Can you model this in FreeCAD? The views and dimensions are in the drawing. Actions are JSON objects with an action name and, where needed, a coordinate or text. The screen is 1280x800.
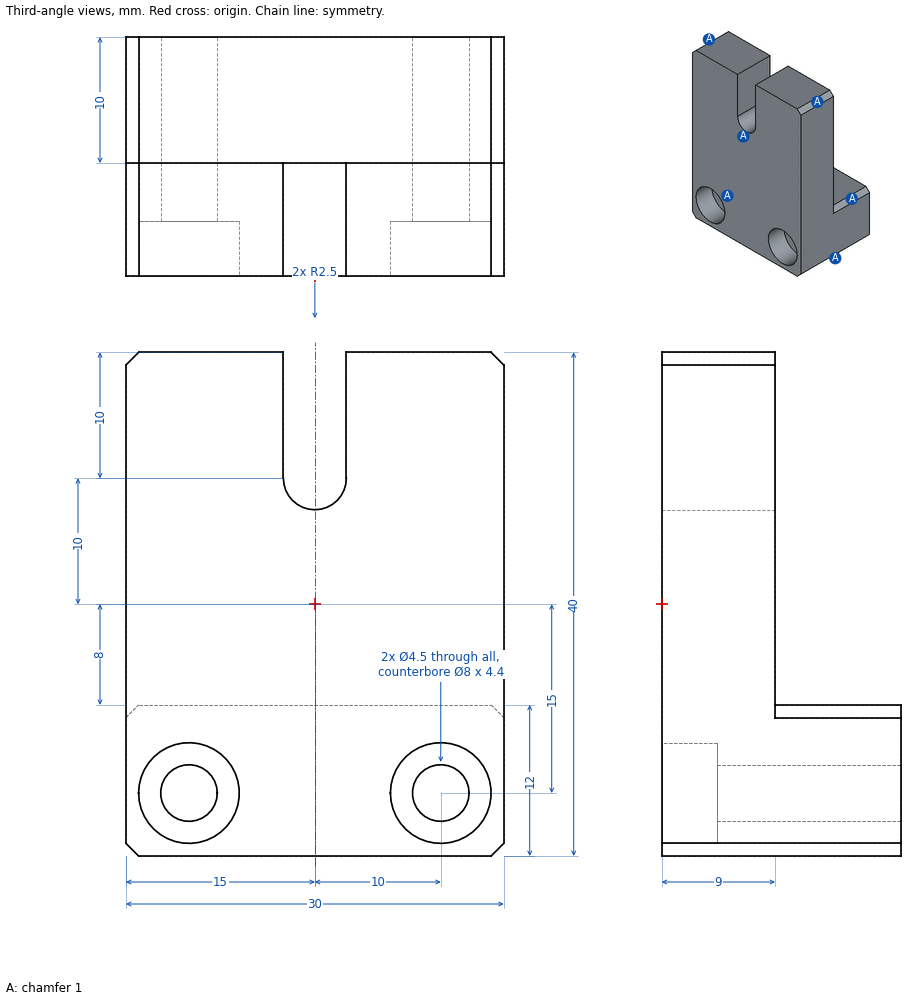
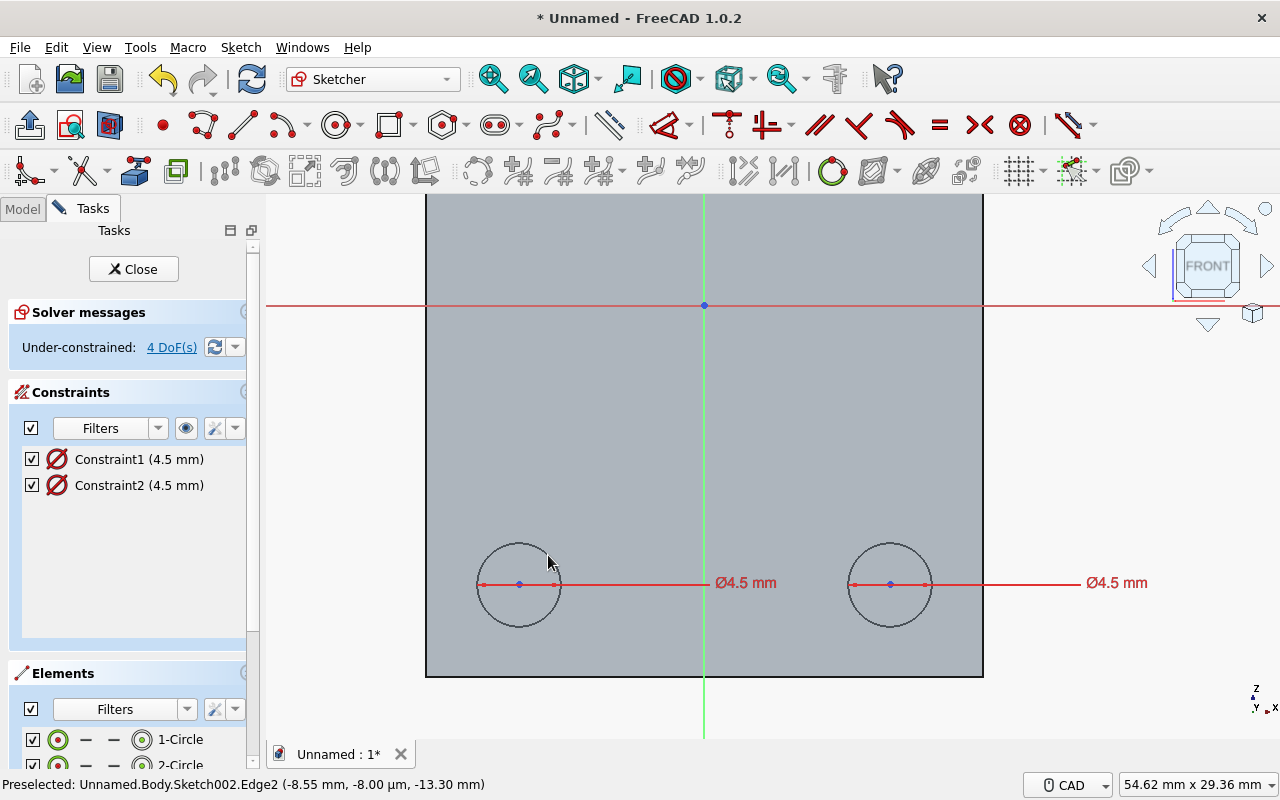
{"action": "left_click", "coordinate": [890, 585]}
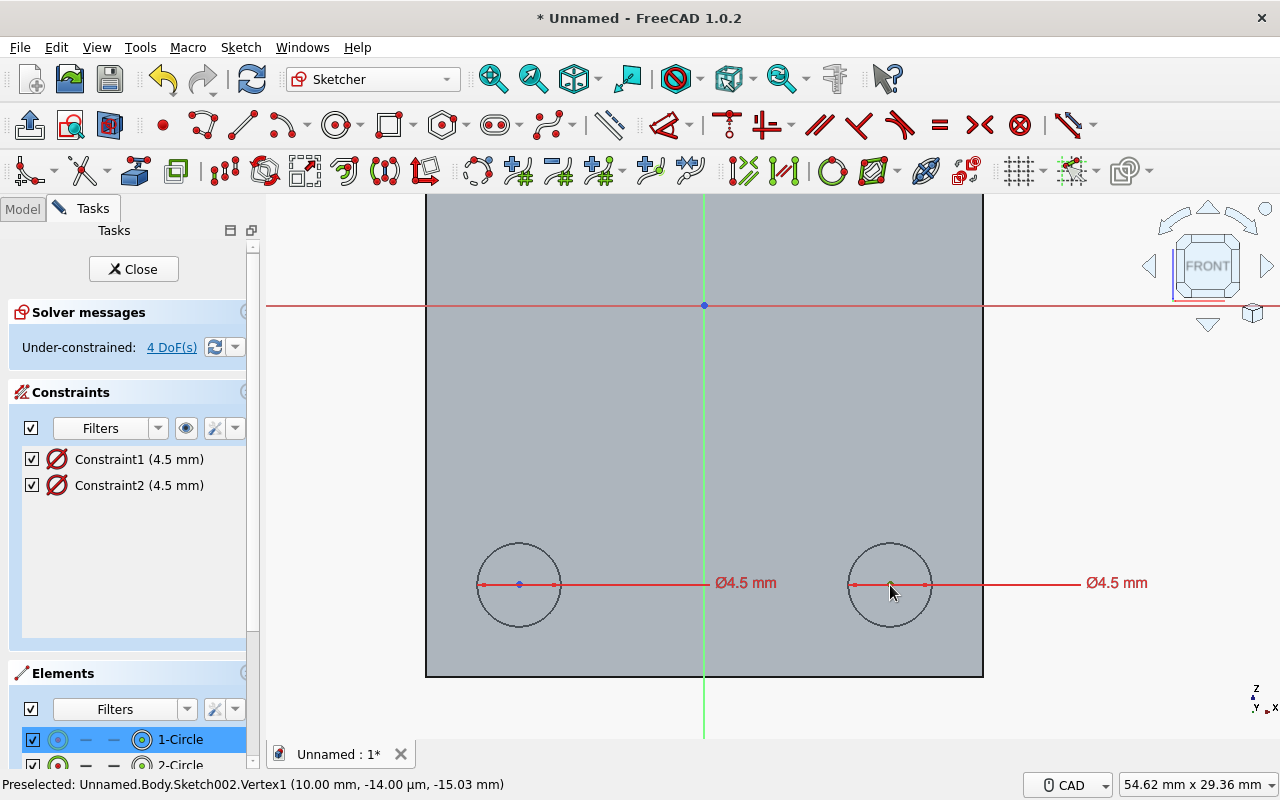
{"action": "left_click", "coordinate": [519, 585]}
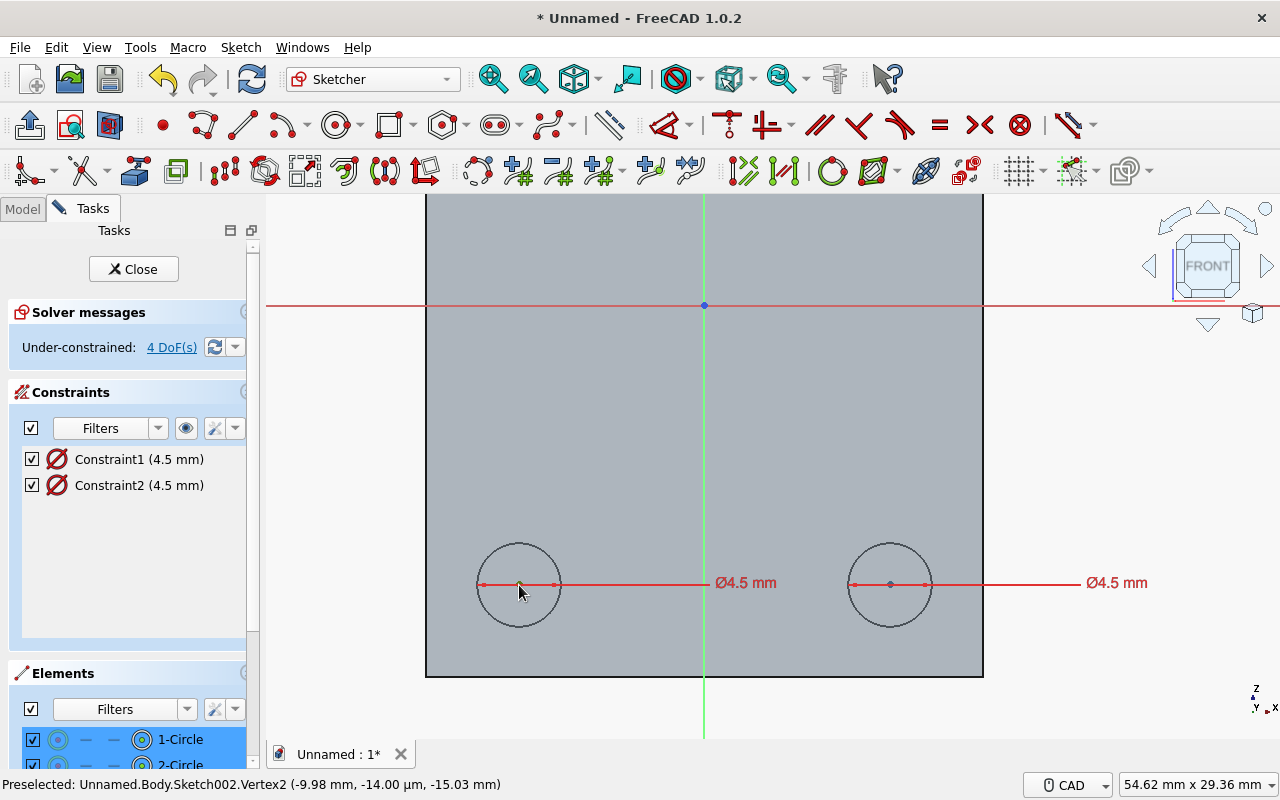
{"action": "left_click", "coordinate": [704, 676]}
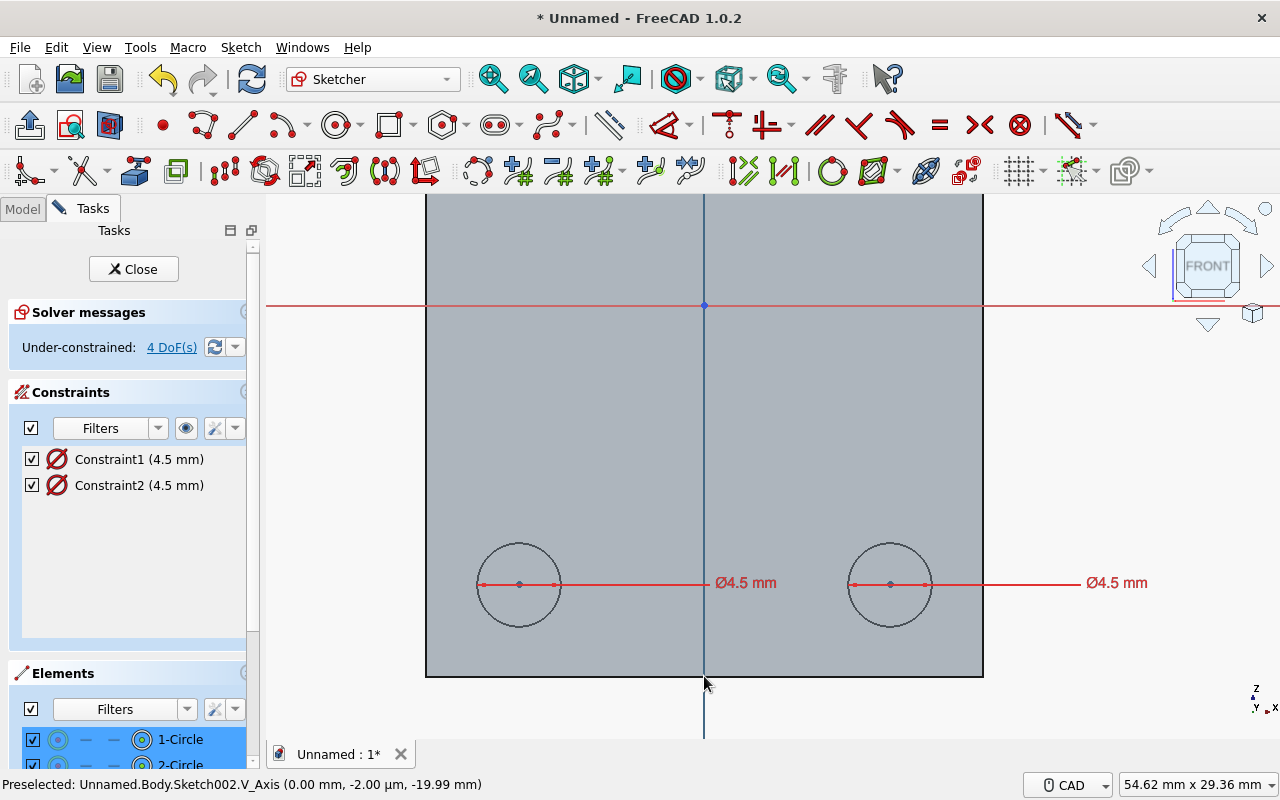
{"action": "left_click", "coordinate": [980, 126]}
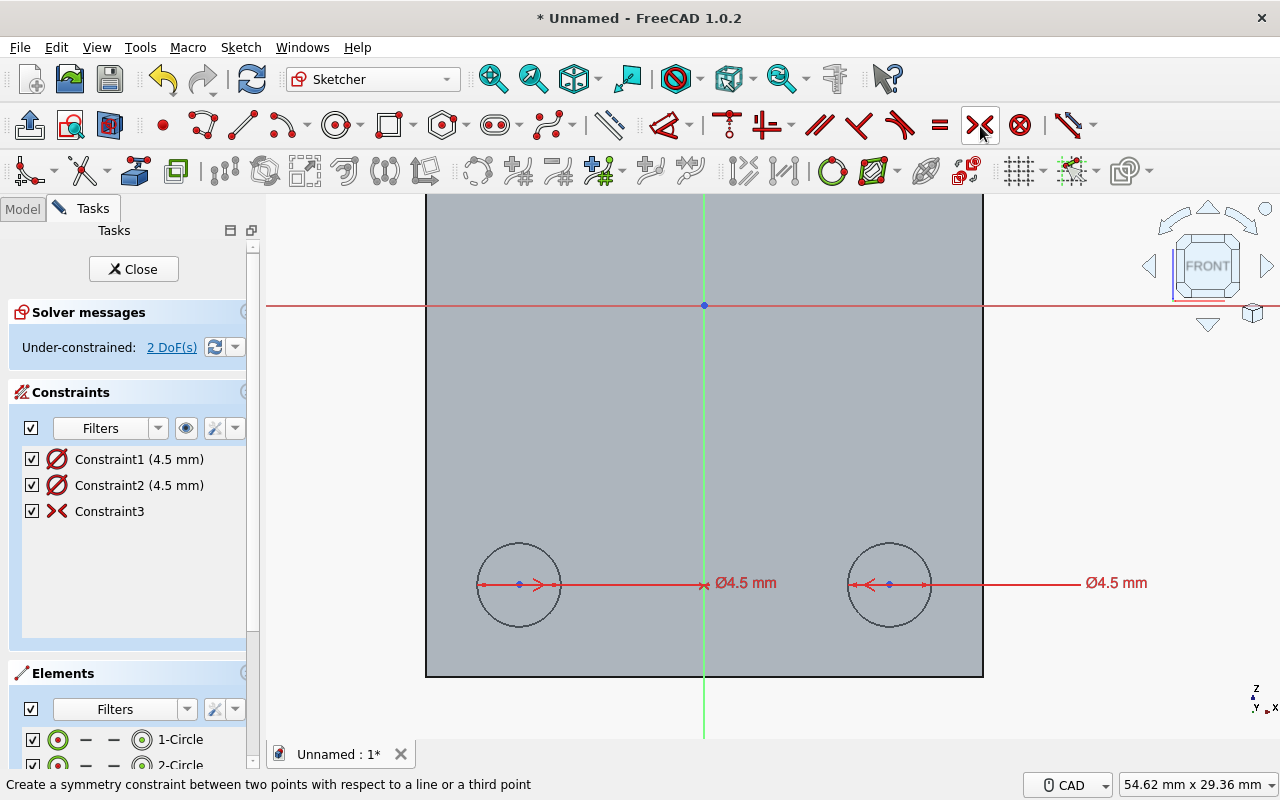
{"action": "left_click", "coordinate": [664, 126]}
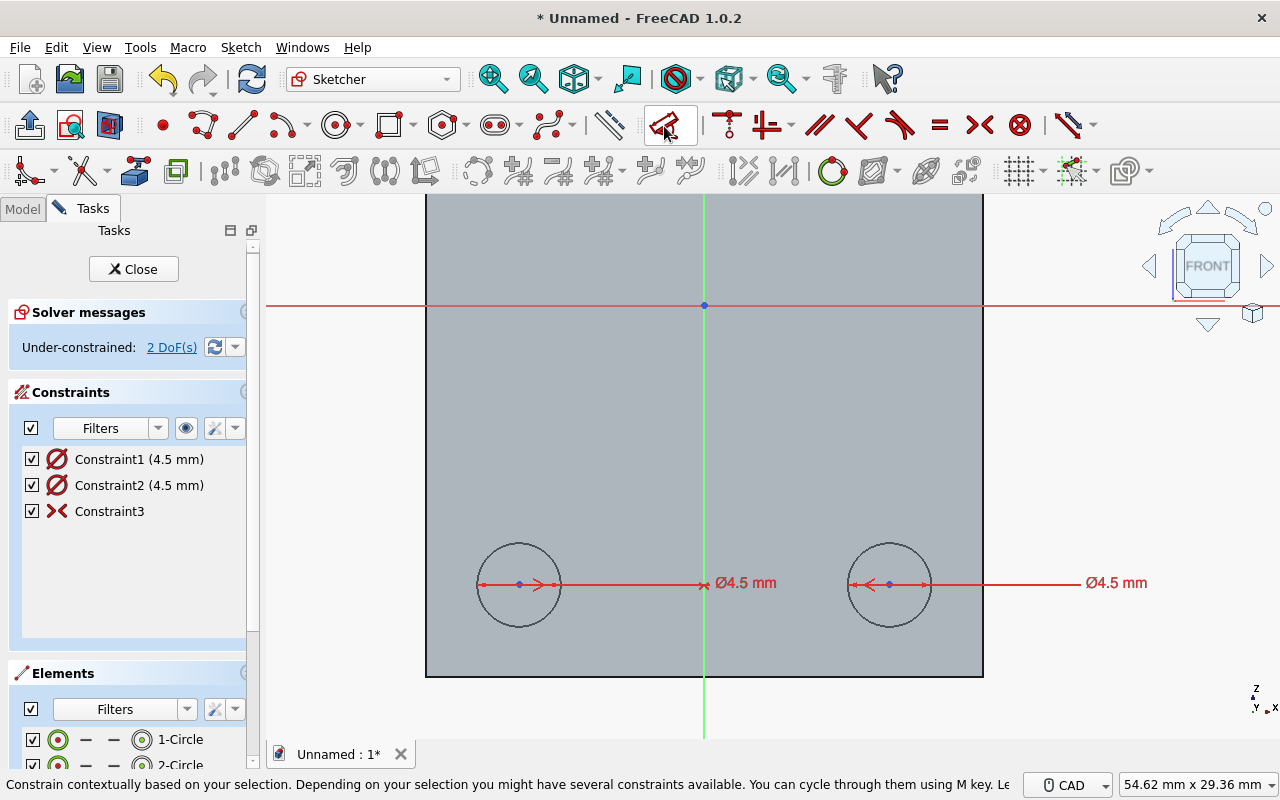
{"action": "left_click", "coordinate": [890, 585]}
{"action": "left_click", "coordinate": [797, 272]}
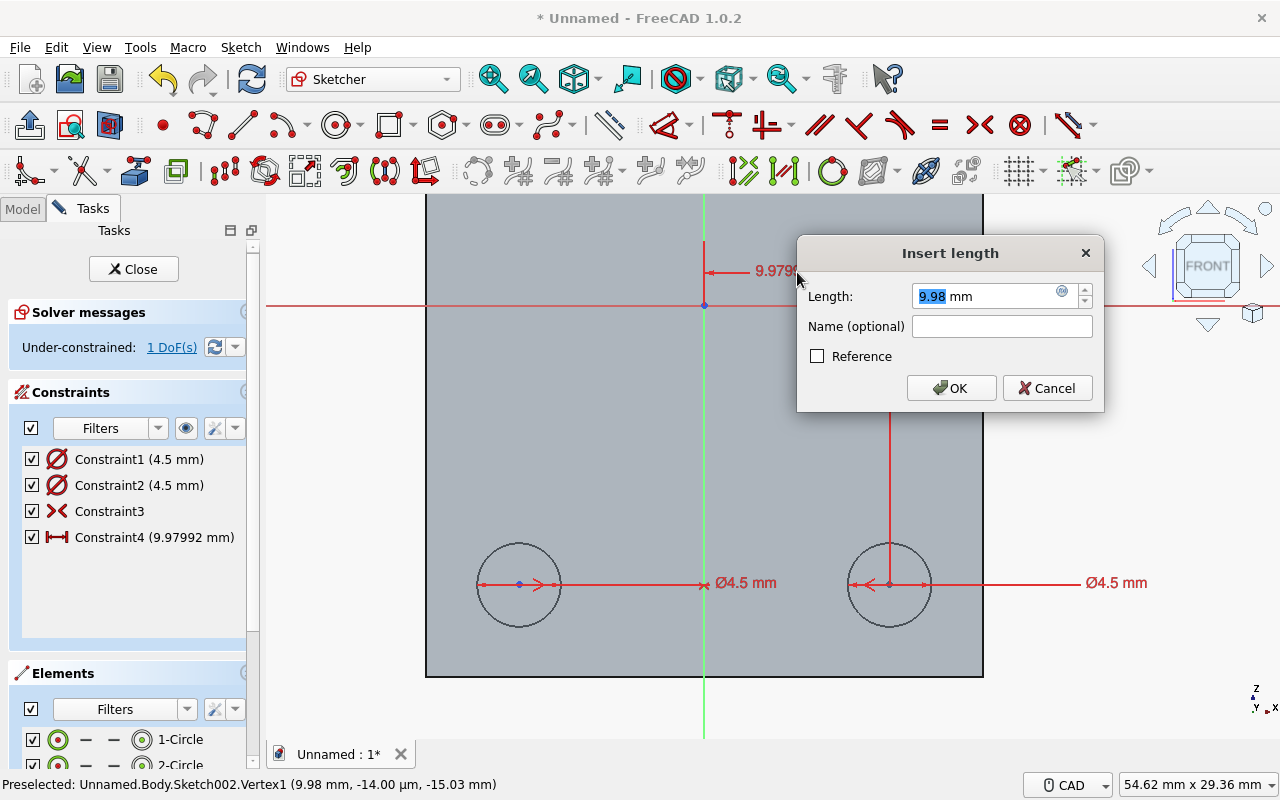
{"action": "type", "text": "10"}
{"action": "key", "text": "Return"}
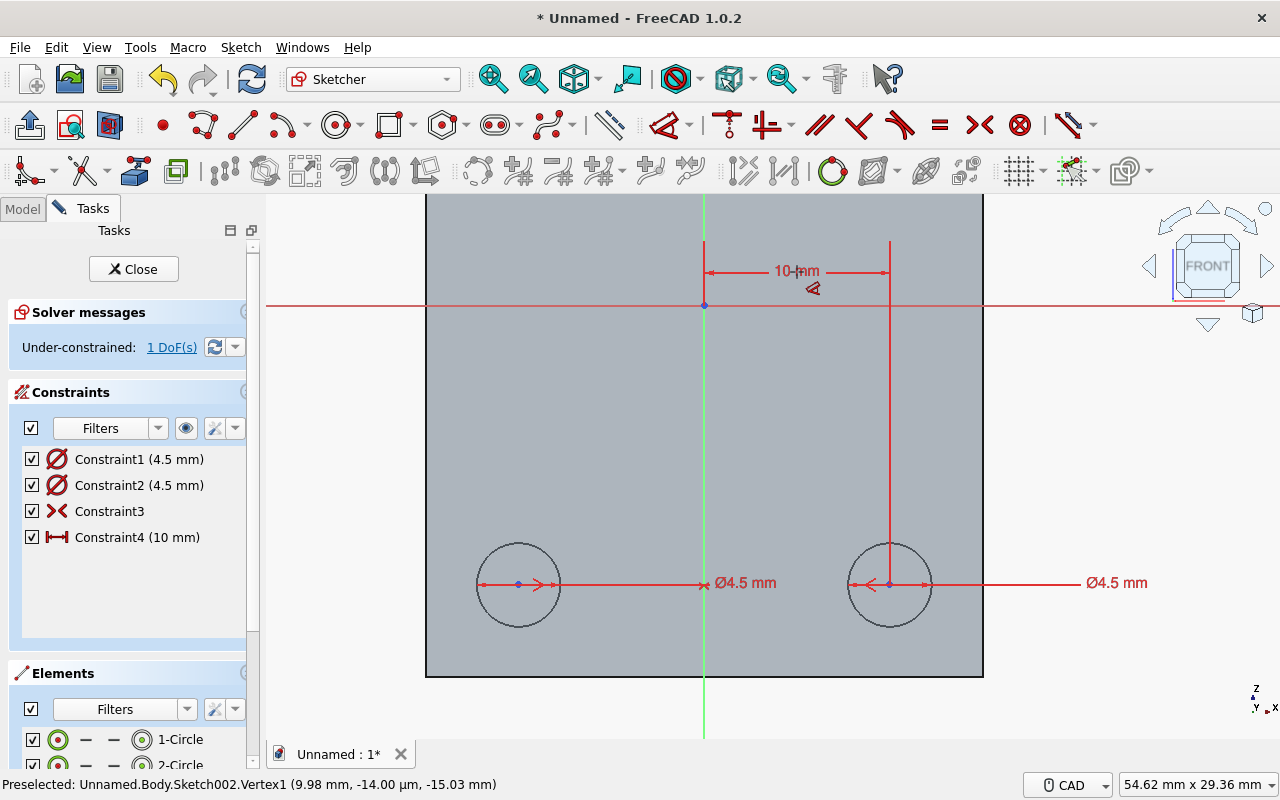
{"action": "left_click", "coordinate": [890, 585]}
{"action": "left_click", "coordinate": [924, 445]}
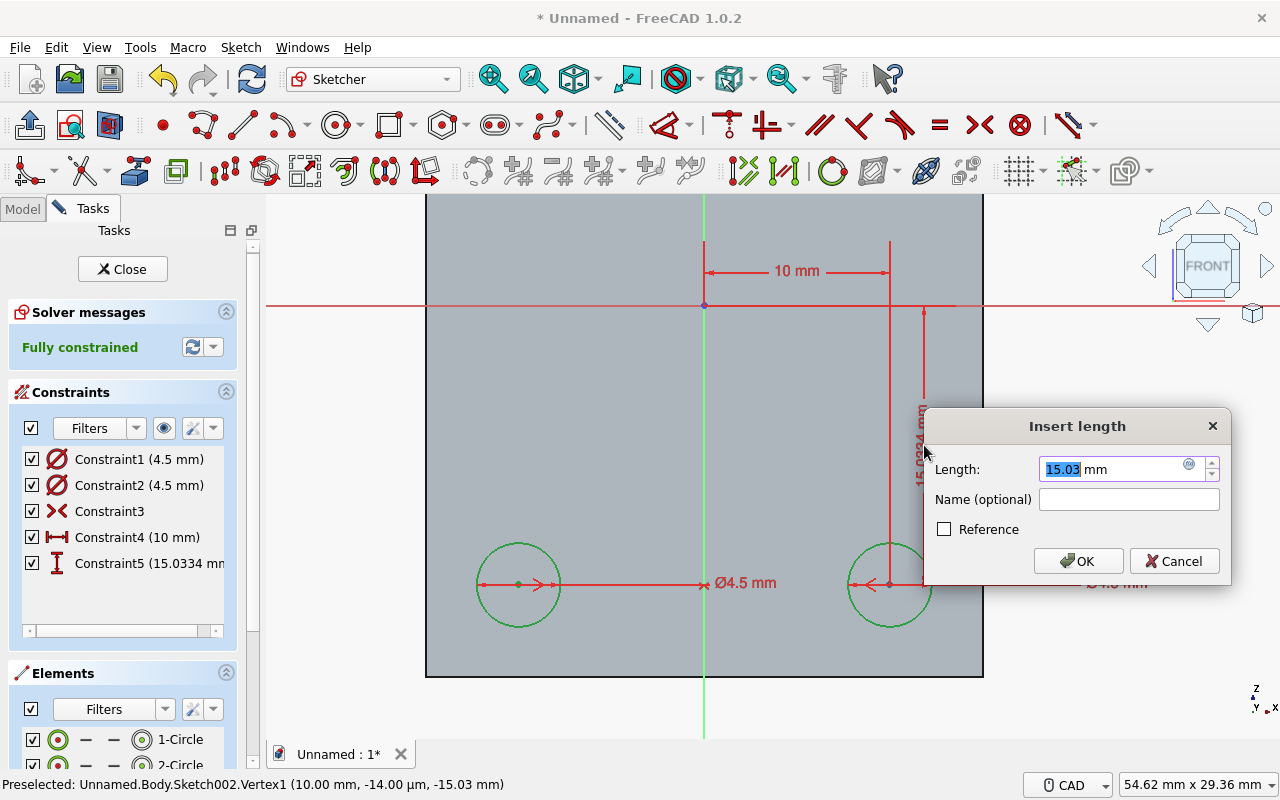
{"action": "type", "text": "15"}
{"action": "key", "text": "Return"}
{"action": "key", "text": "Escape"}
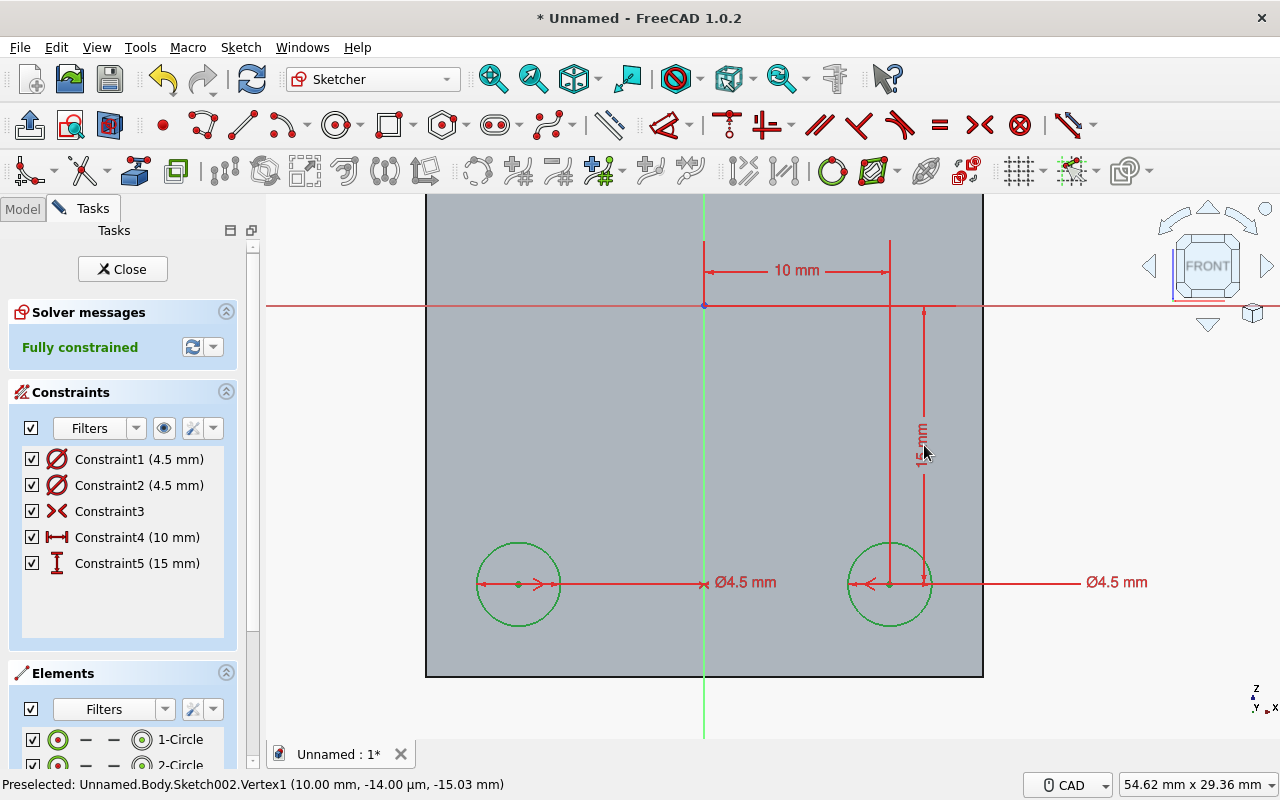
{"action": "left_click", "coordinate": [123, 269]}